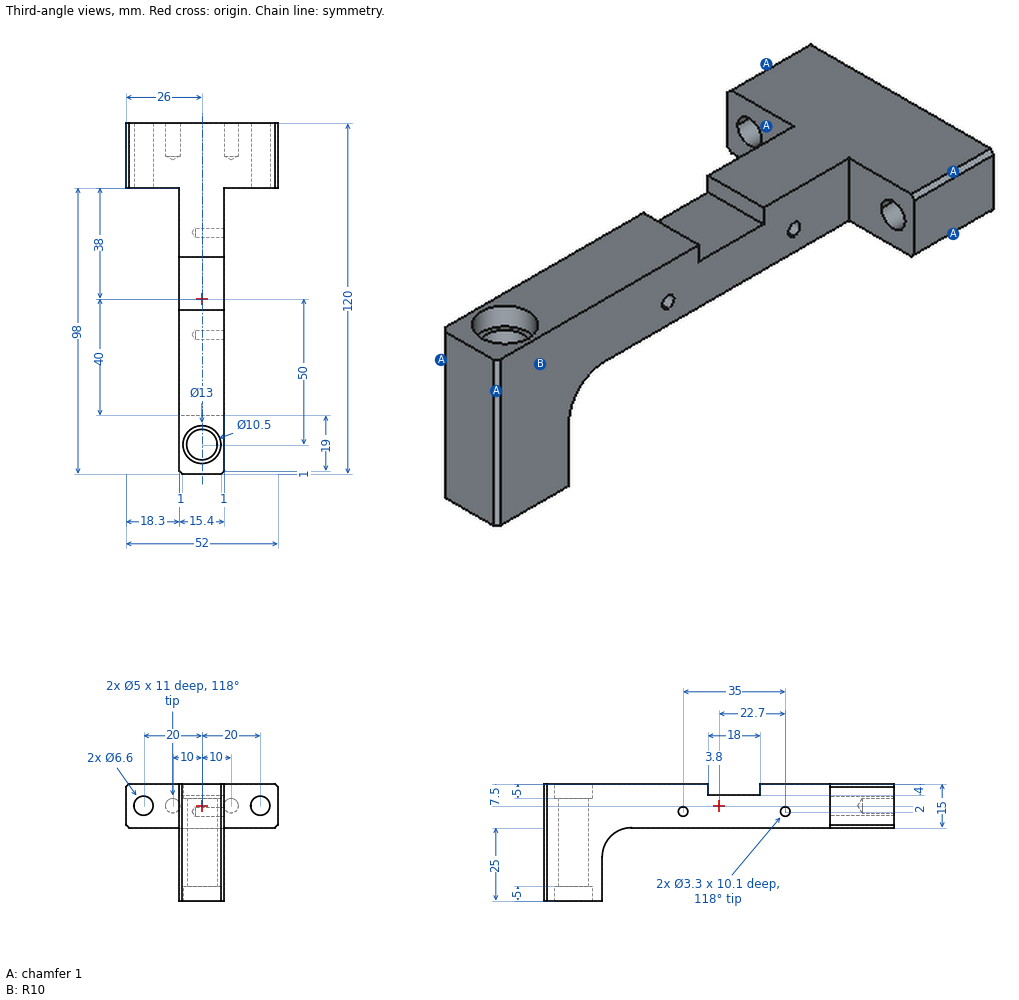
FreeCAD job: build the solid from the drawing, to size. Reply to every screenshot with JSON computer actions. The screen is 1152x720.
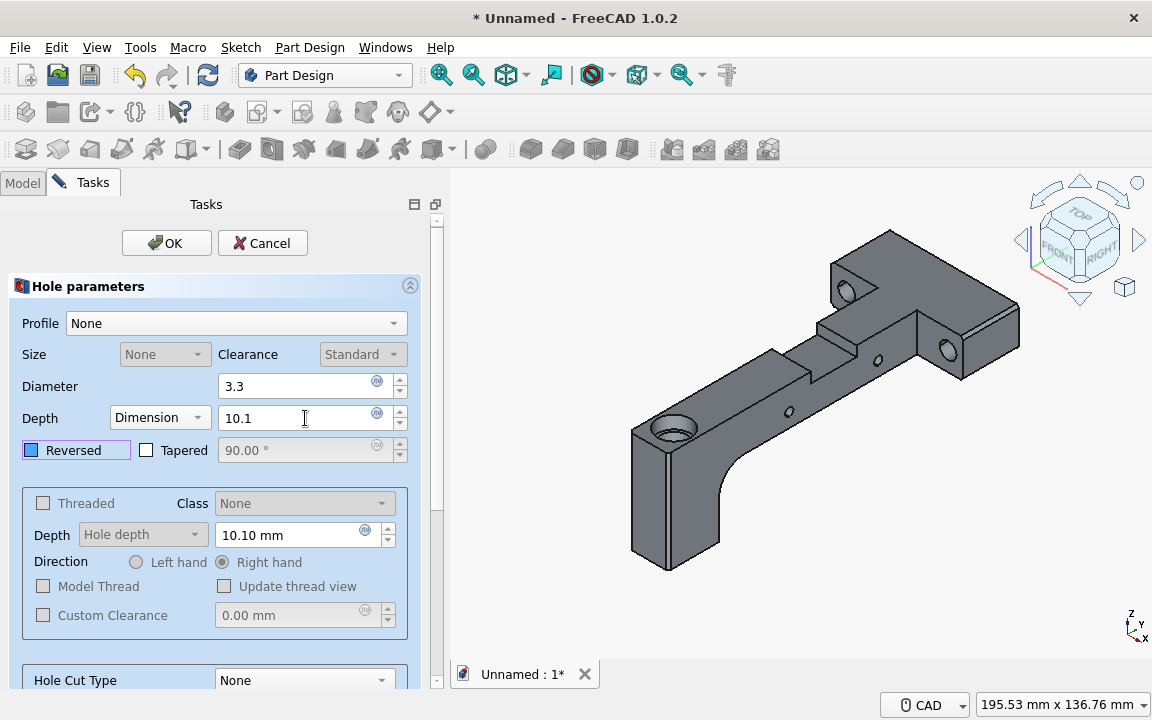
{"action": "left_click", "coordinate": [167, 243]}